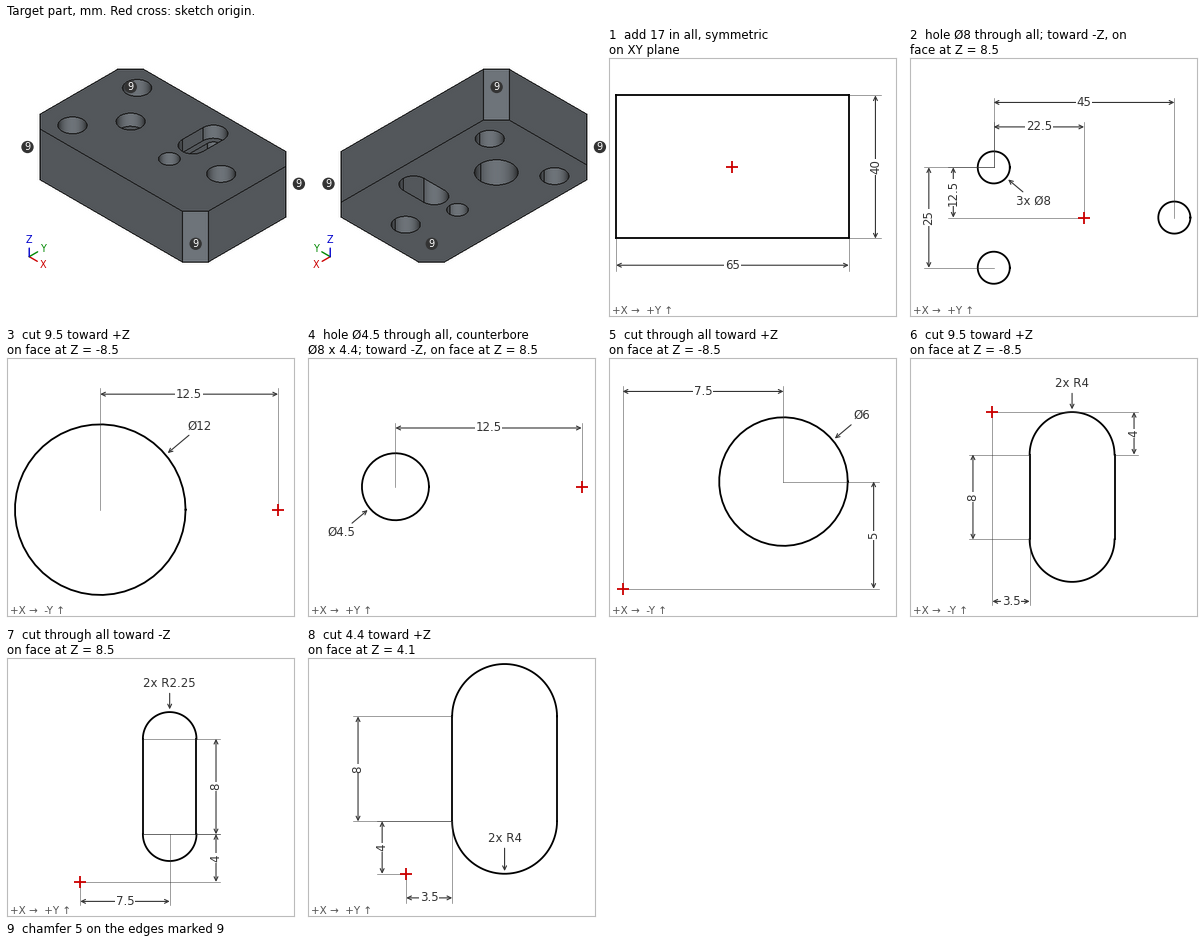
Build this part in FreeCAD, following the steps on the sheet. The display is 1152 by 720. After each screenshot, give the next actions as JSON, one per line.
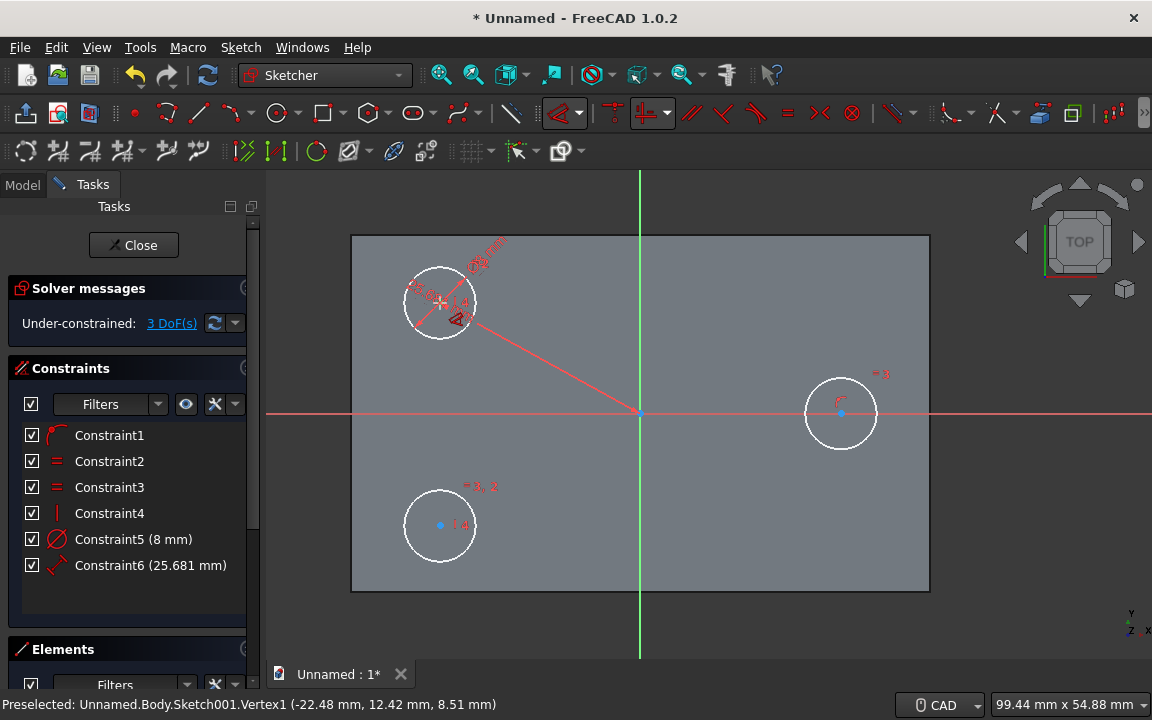
{"action": "left_click", "coordinate": [440, 526]}
{"action": "left_click", "coordinate": [406, 363]}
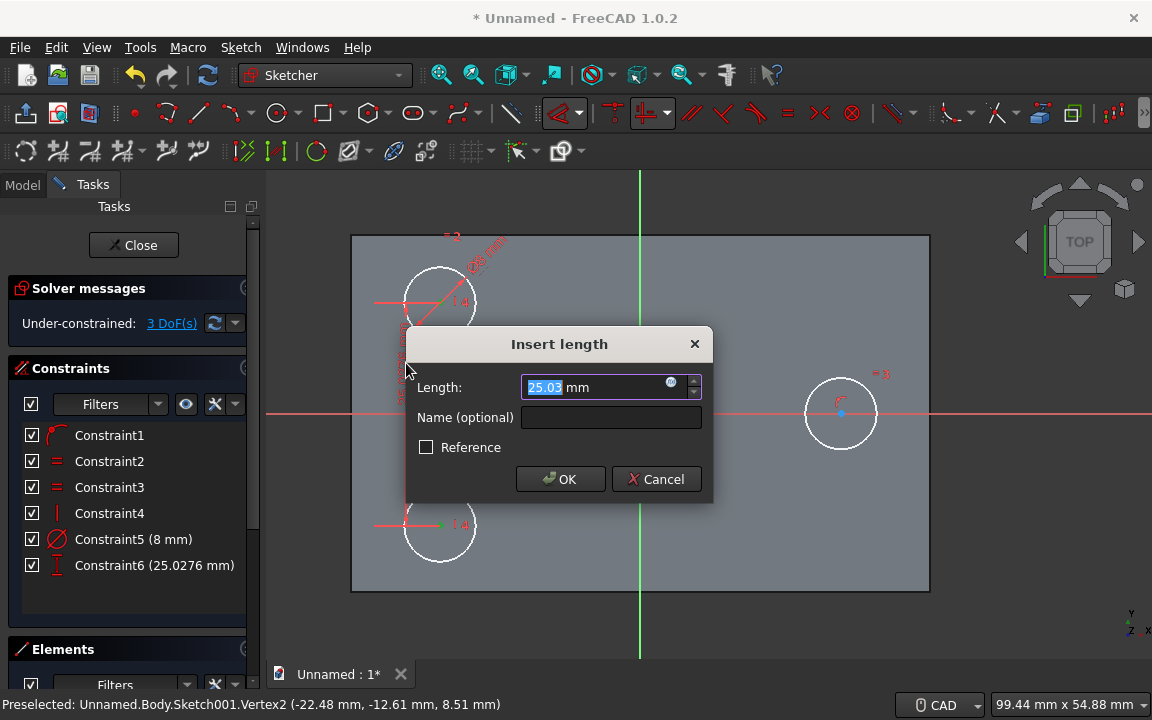
{"action": "type", "text": "25"}
{"action": "key", "text": "Return"}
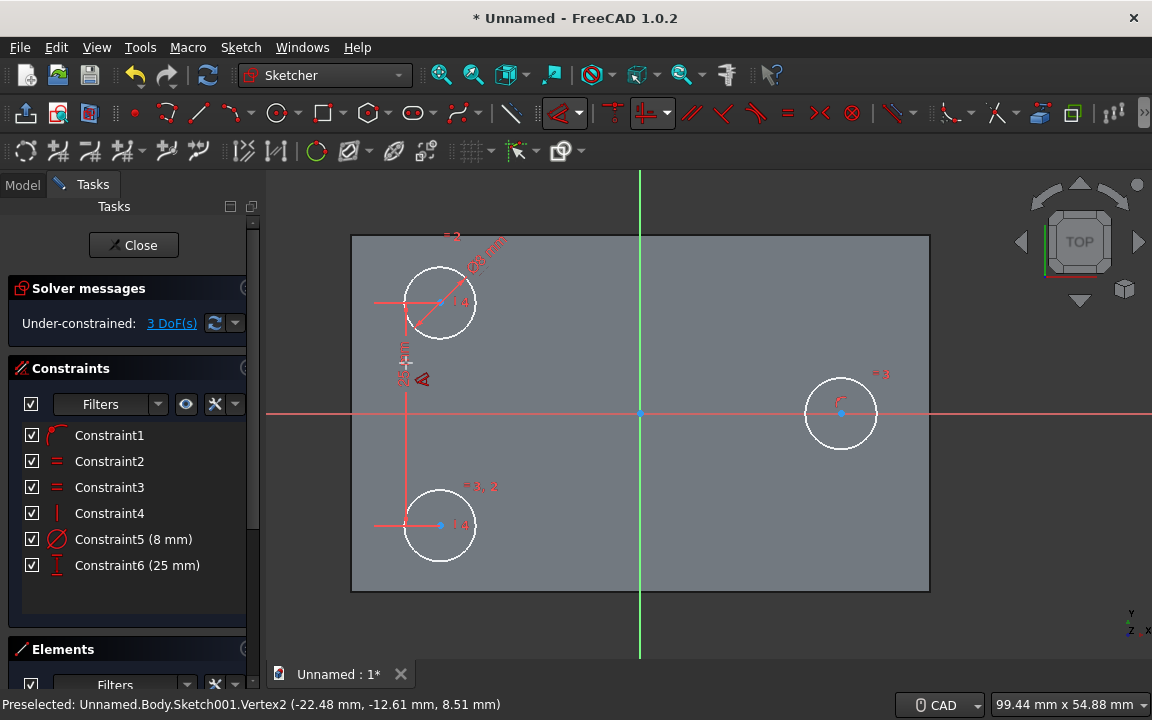
{"action": "left_click", "coordinate": [440, 303]}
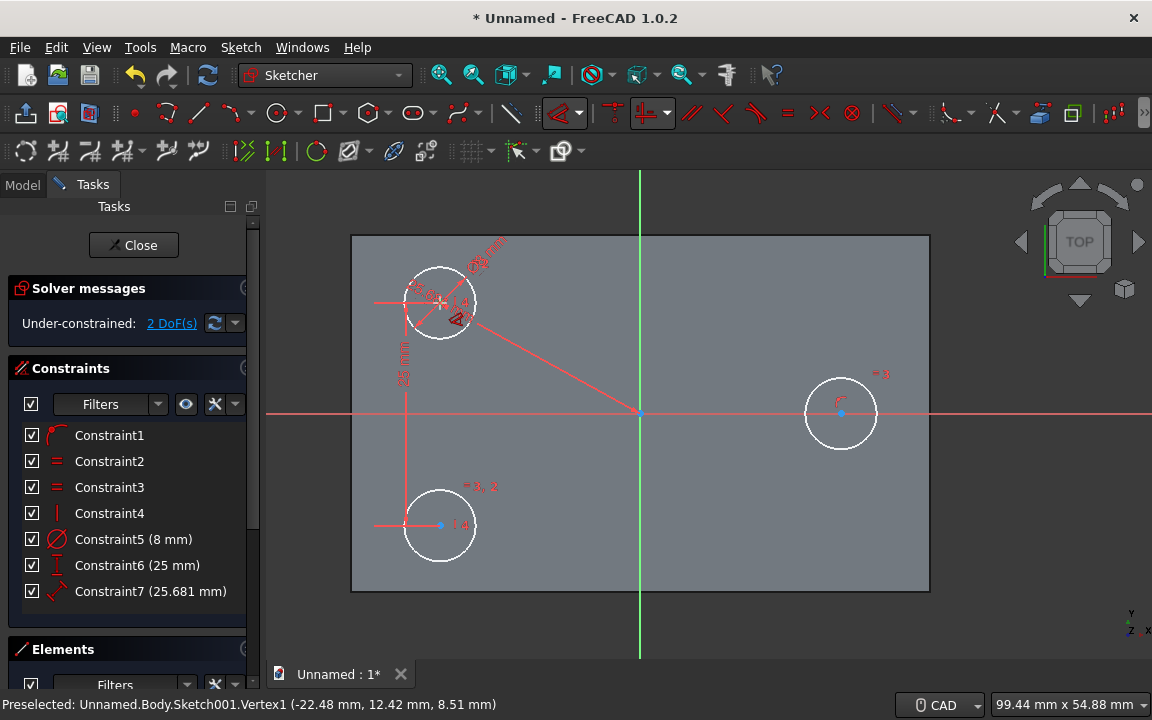
{"action": "left_click", "coordinate": [841, 414]}
{"action": "left_click", "coordinate": [733, 269]}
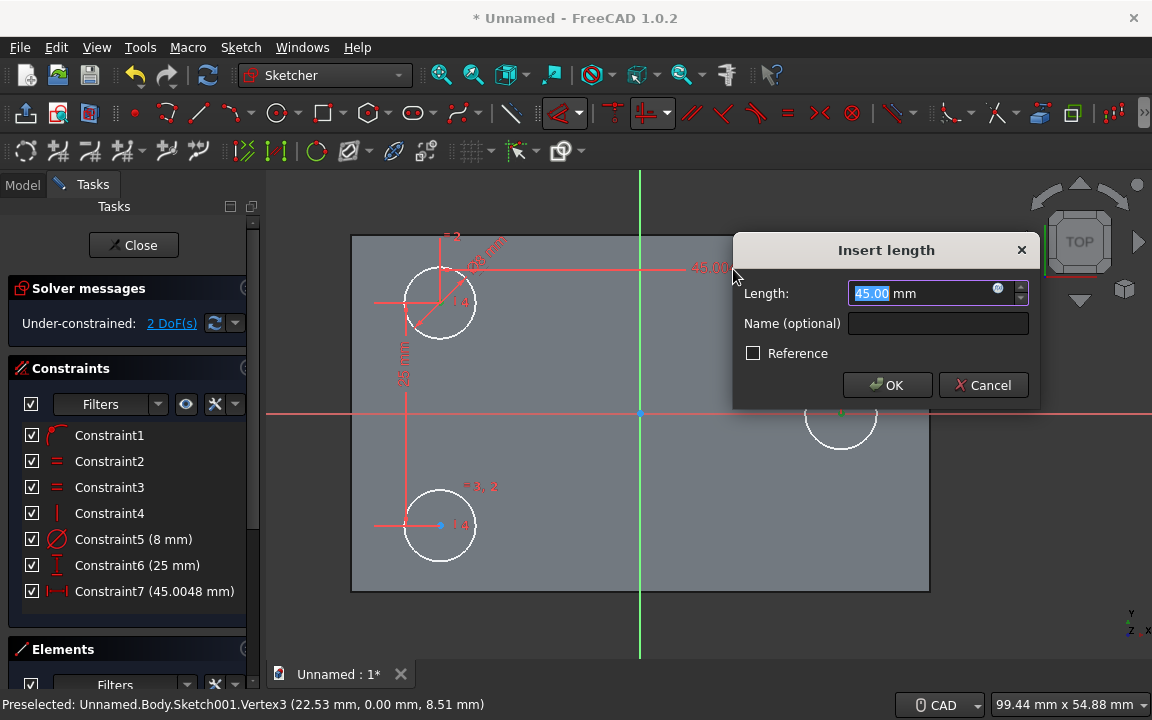
{"action": "type", "text": "45"}
{"action": "key", "text": "Return"}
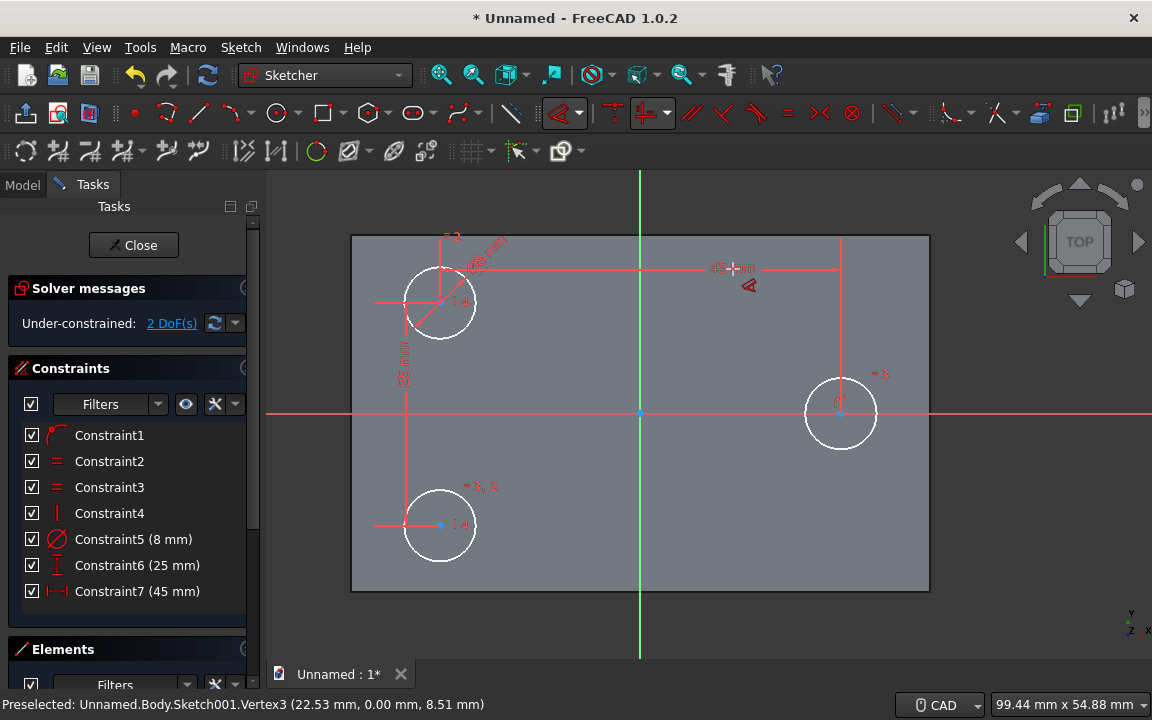
{"action": "left_click", "coordinate": [440, 303]}
{"action": "left_click", "coordinate": [586, 269]}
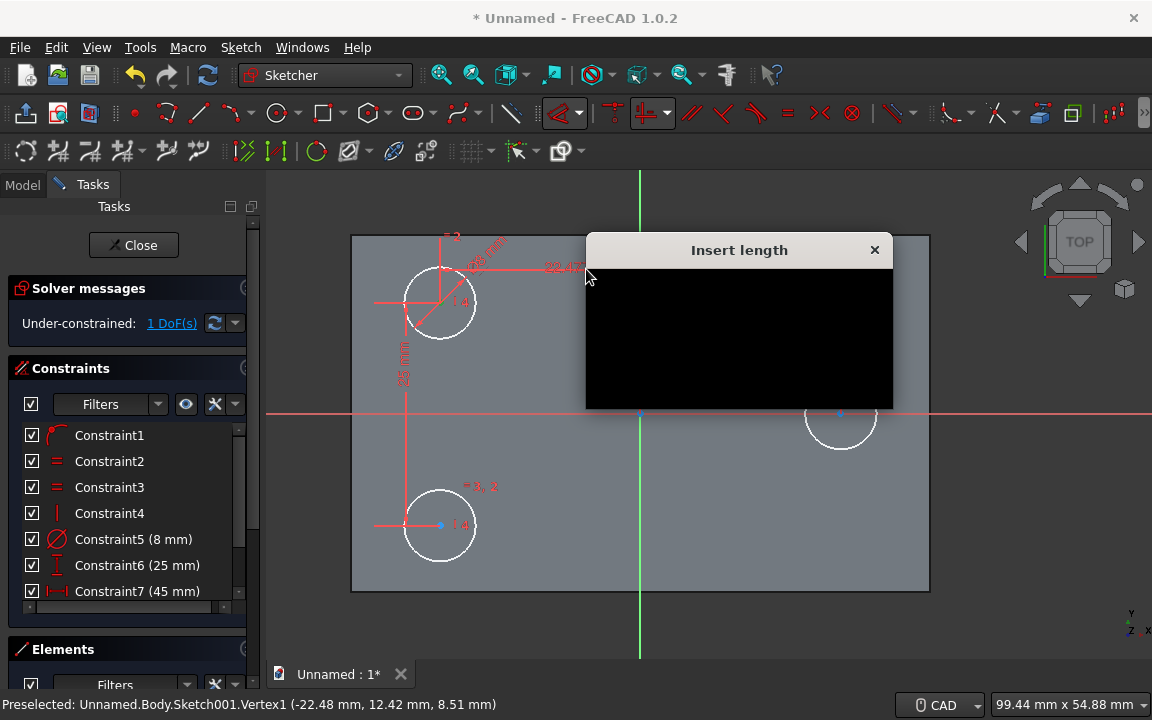
{"action": "type", "text": "22.5"}
{"action": "key", "text": "Return"}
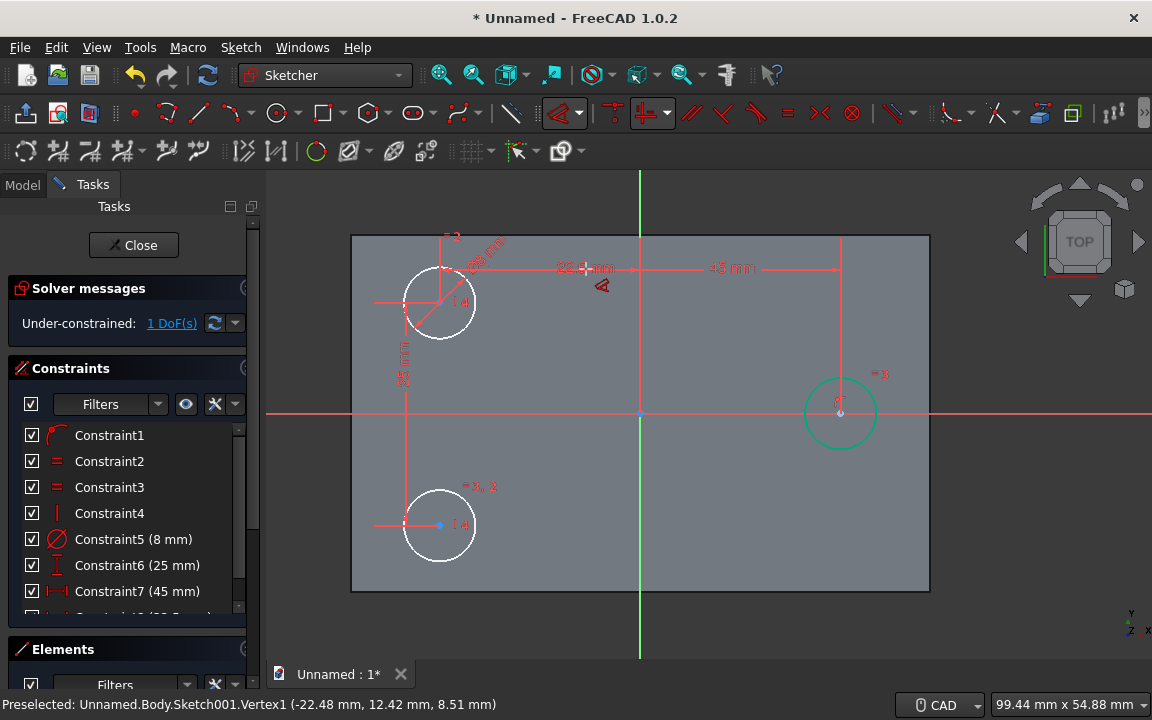
{"action": "left_click", "coordinate": [440, 303]}
{"action": "left_click", "coordinate": [406, 384]}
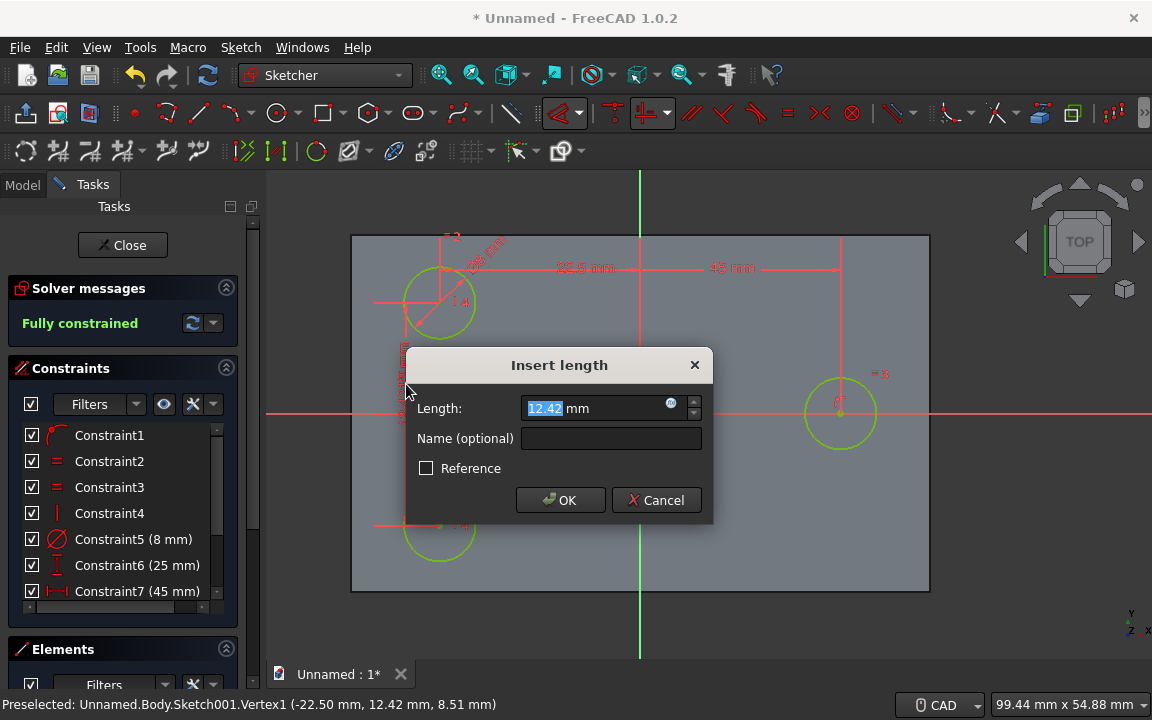
{"action": "type", "text": "12.5"}
{"action": "key", "text": "Return"}
{"action": "key", "text": "Escape"}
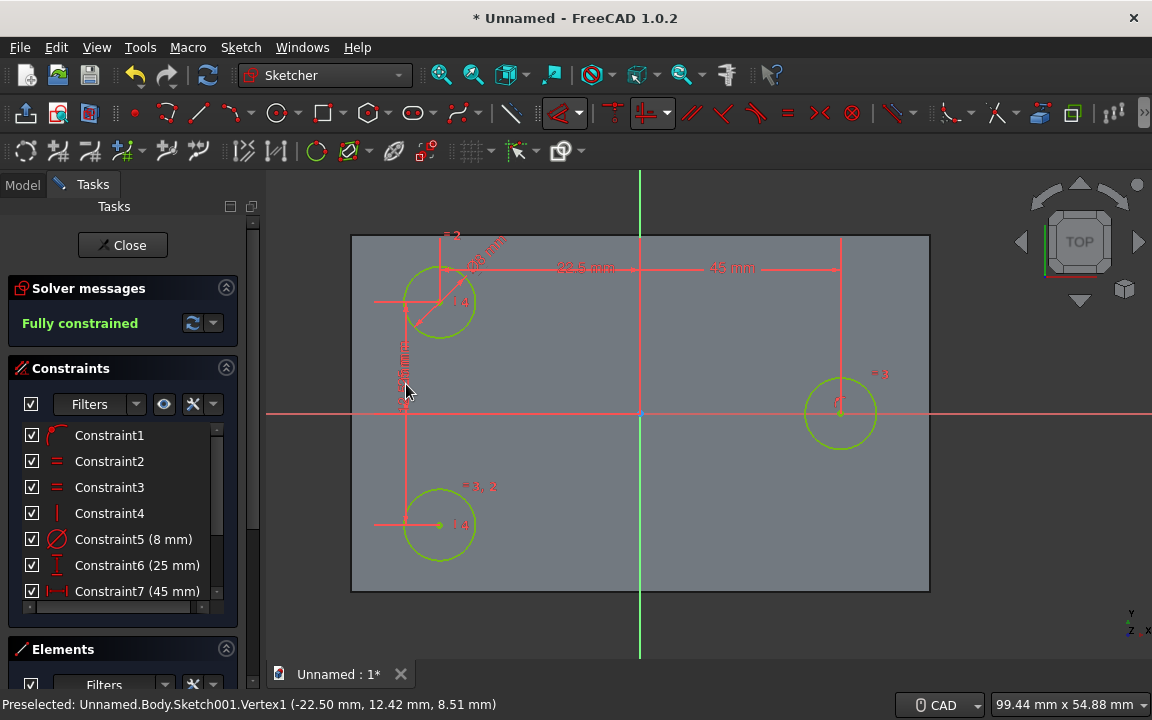
{"action": "left_click", "coordinate": [123, 245]}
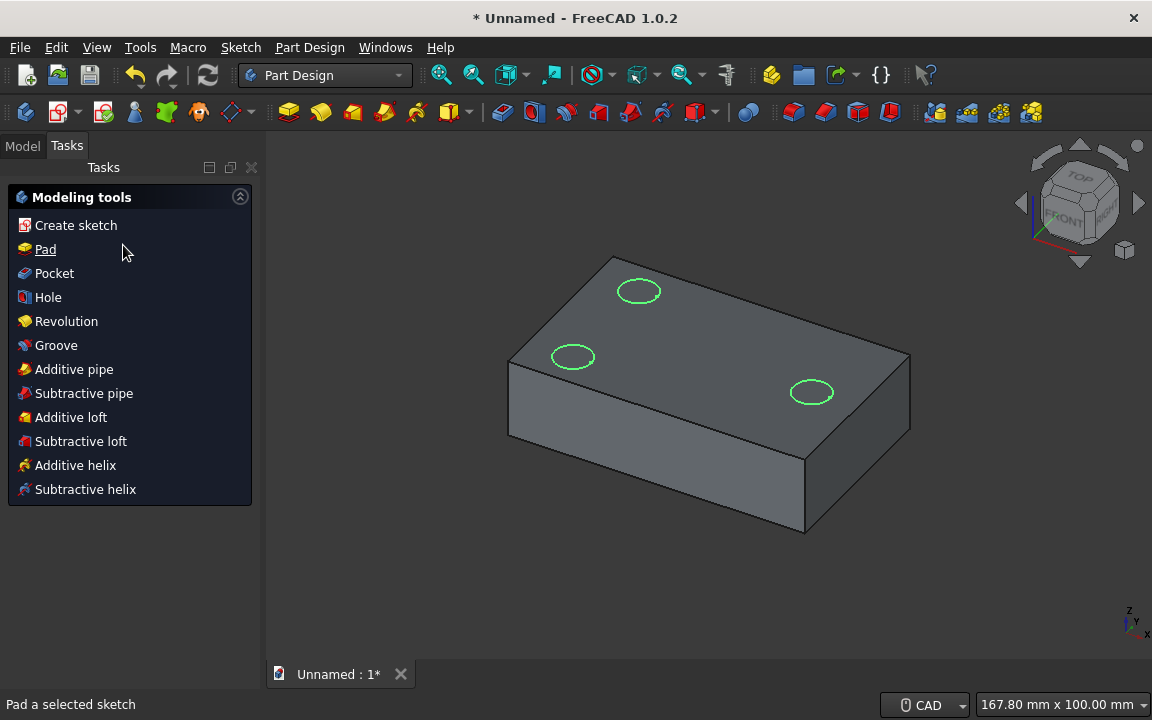
{"action": "left_click", "coordinate": [536, 112]}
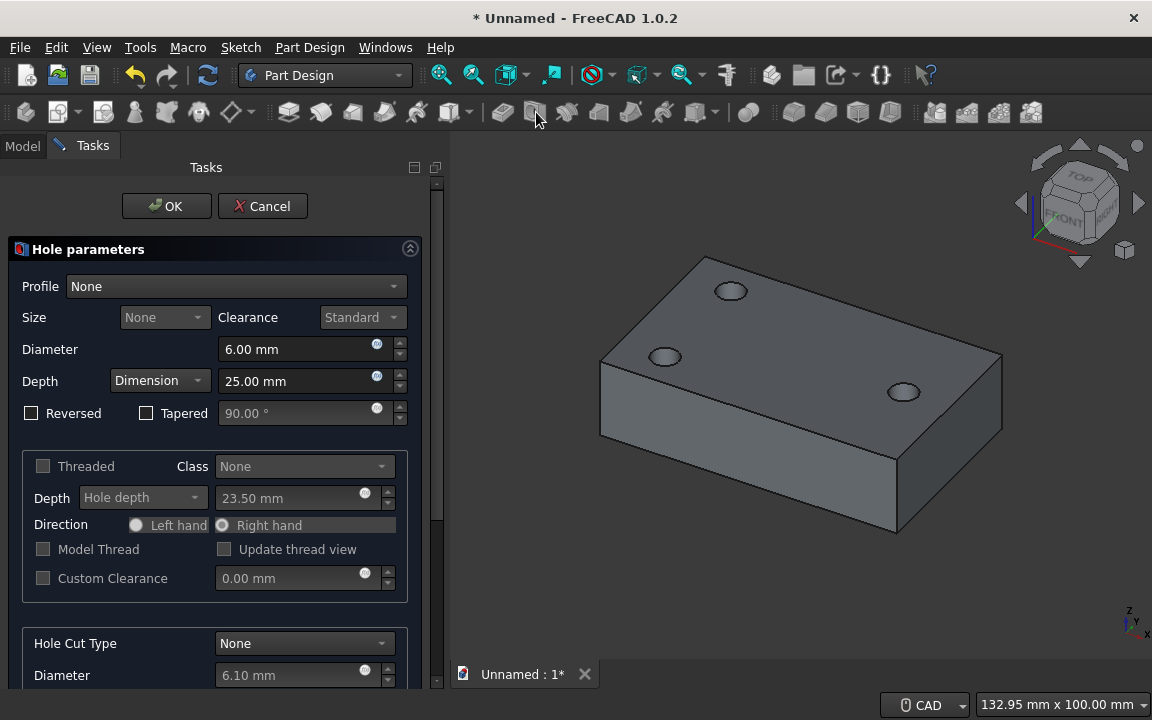
{"action": "triple_click", "coordinate": [305, 349]}